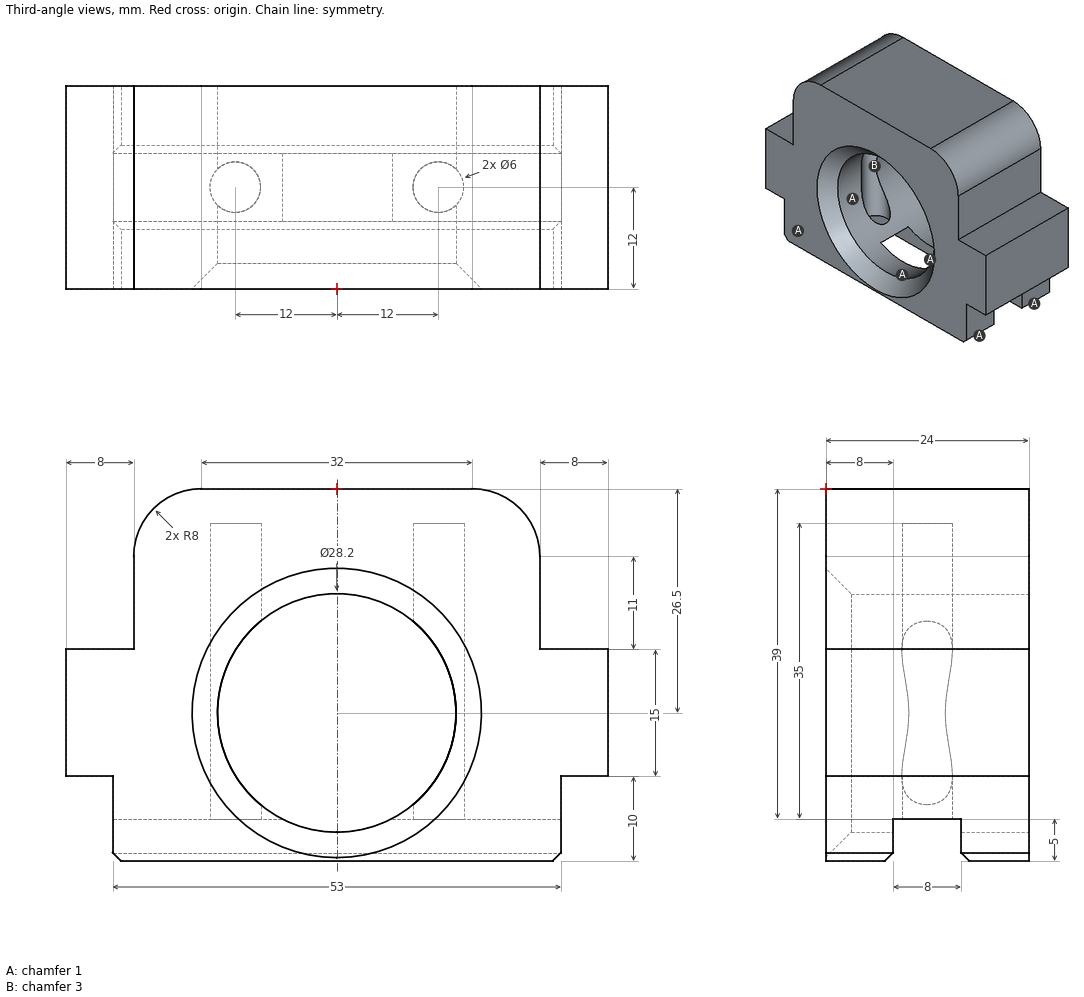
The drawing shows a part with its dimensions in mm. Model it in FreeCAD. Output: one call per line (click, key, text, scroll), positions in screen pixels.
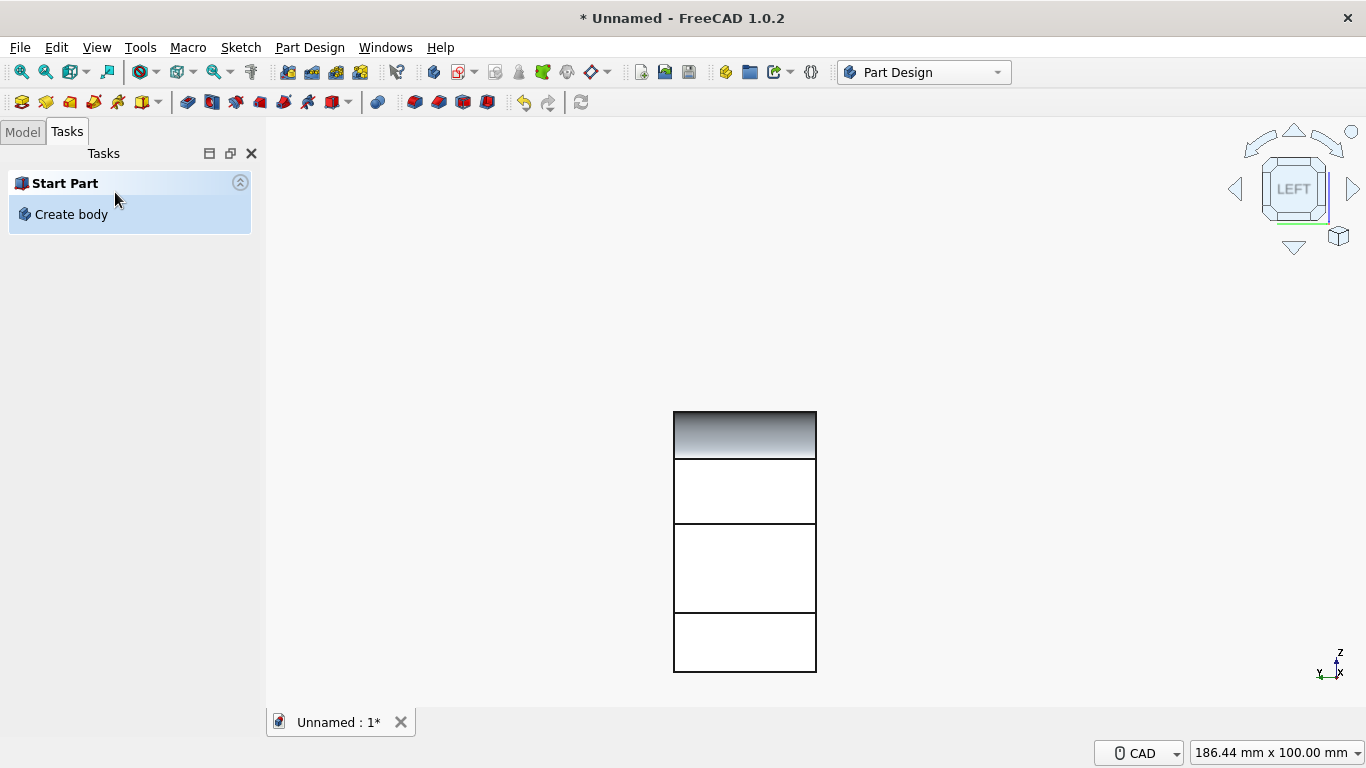
click(22, 72)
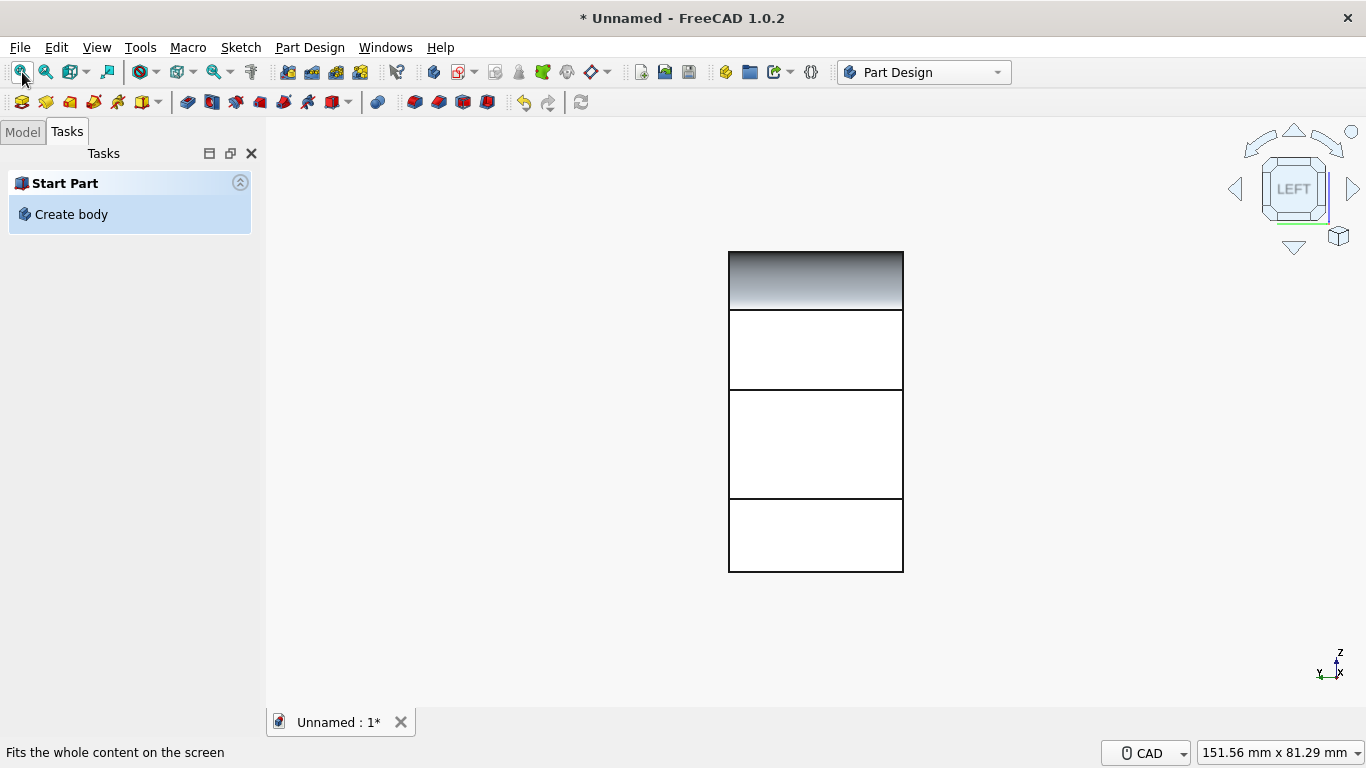
click(766, 534)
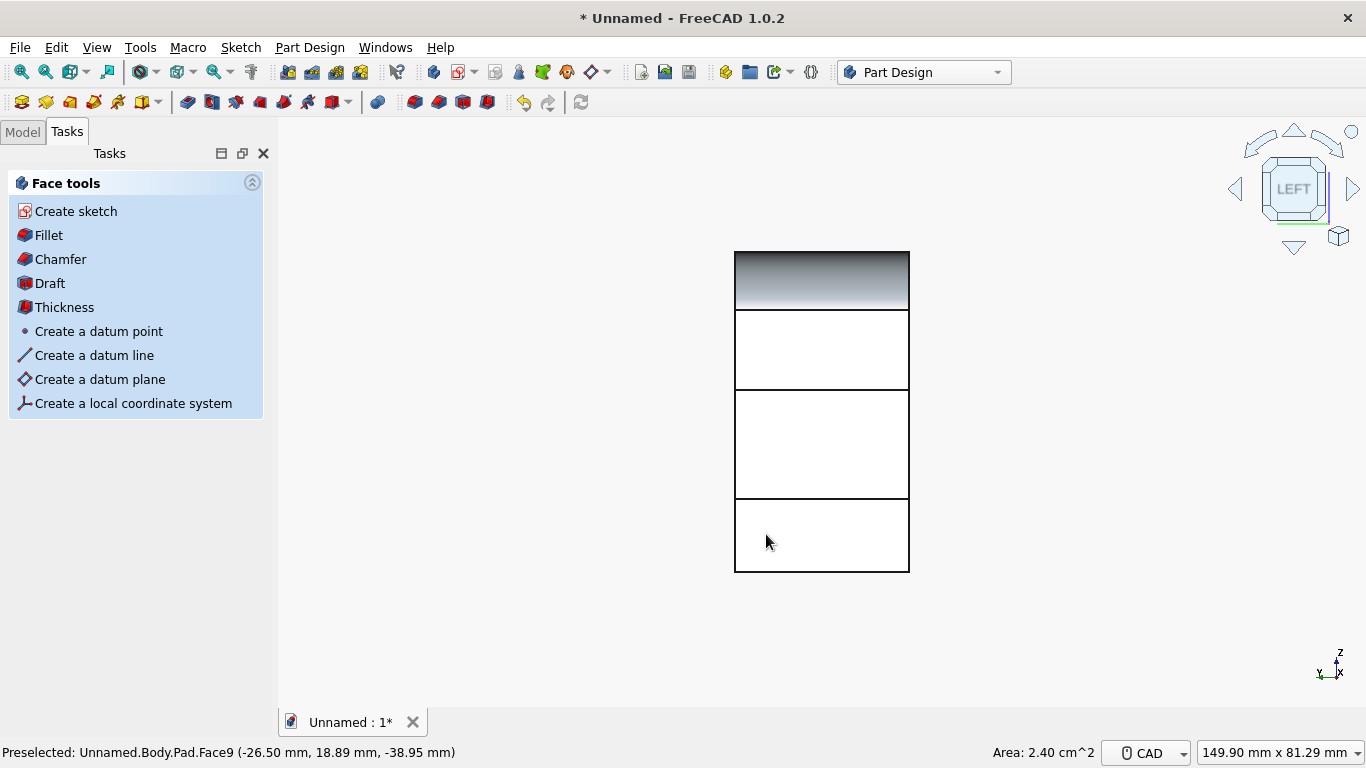
click(458, 72)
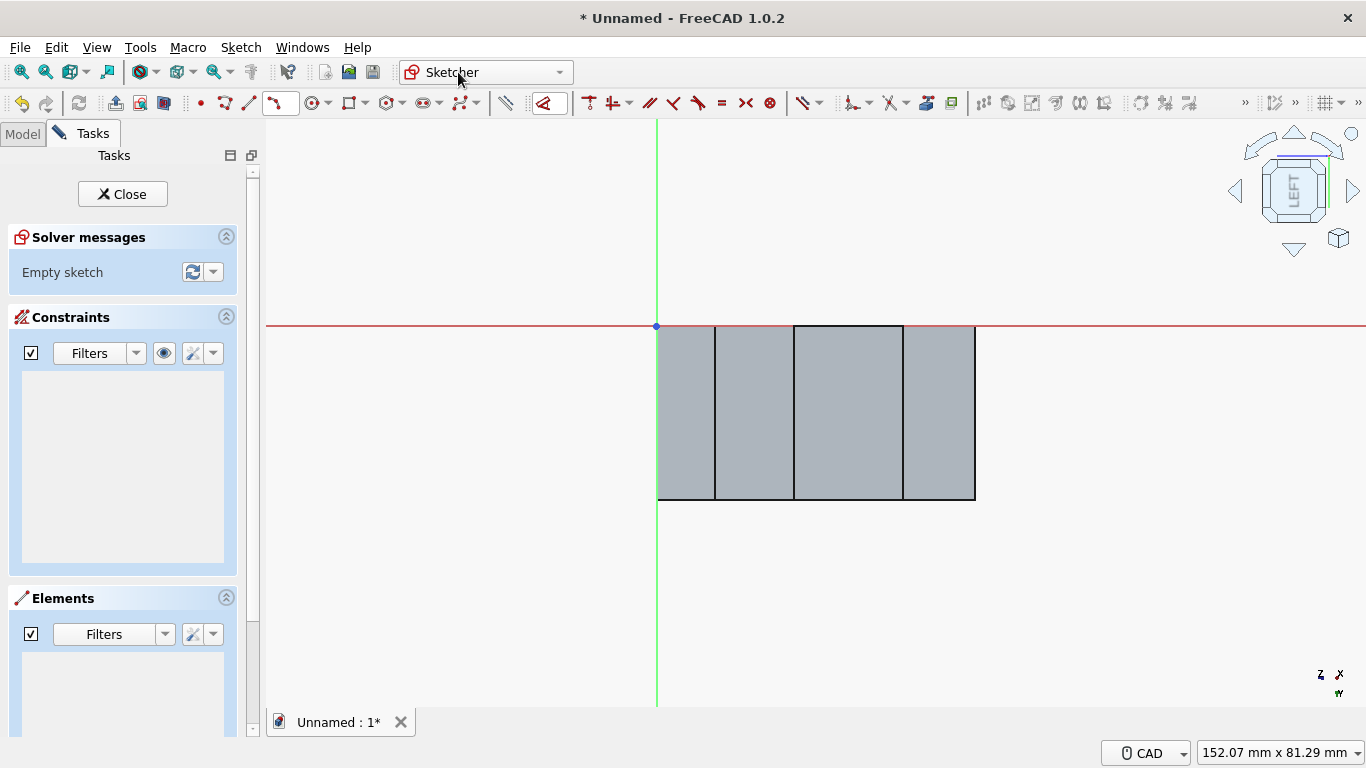
click(164, 104)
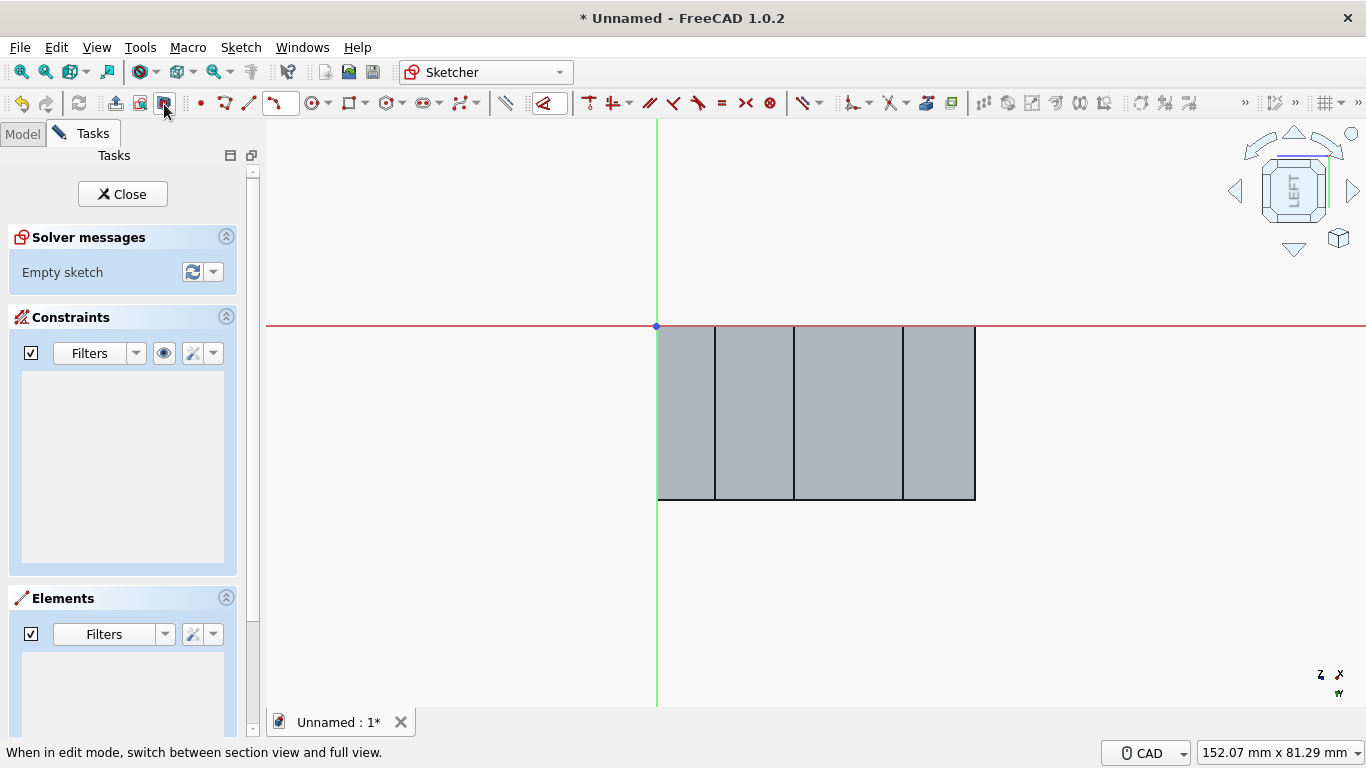
scroll(999, 413, up, 9)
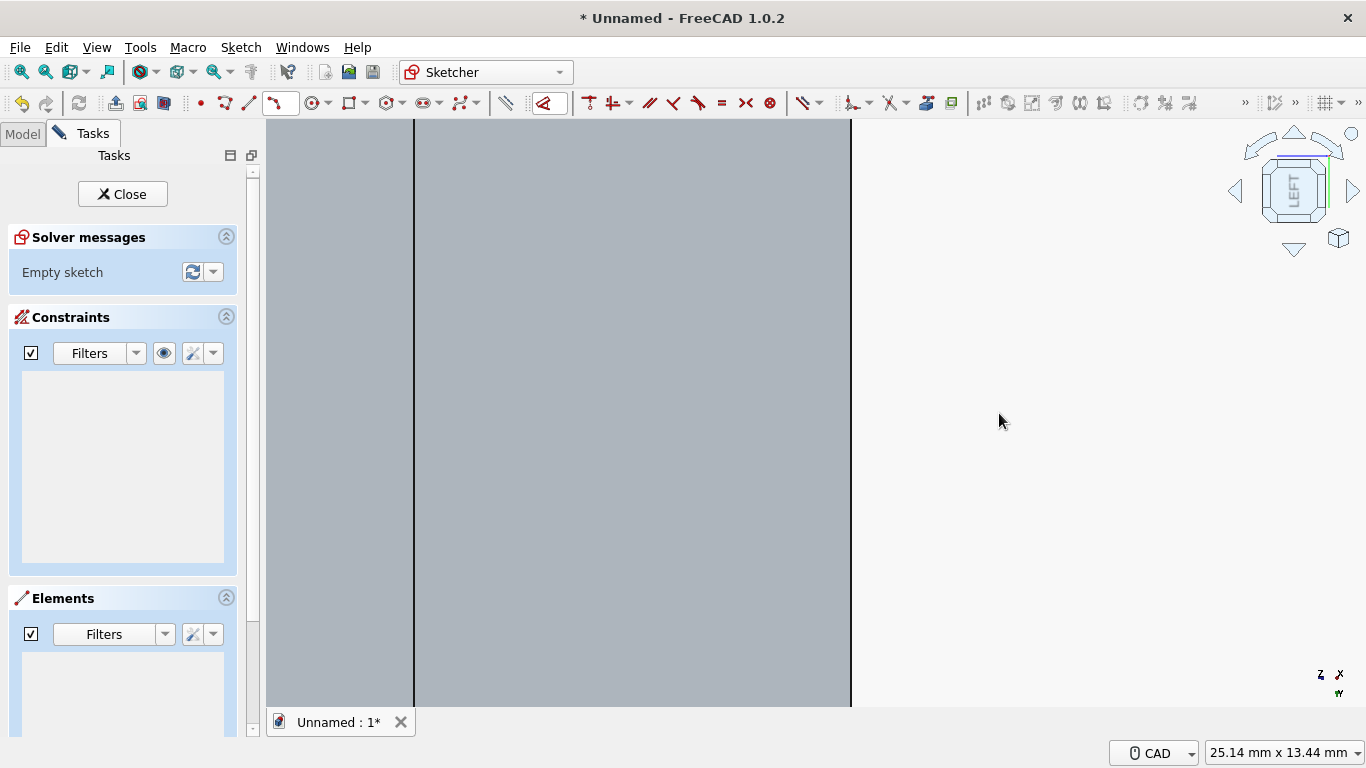
click(350, 104)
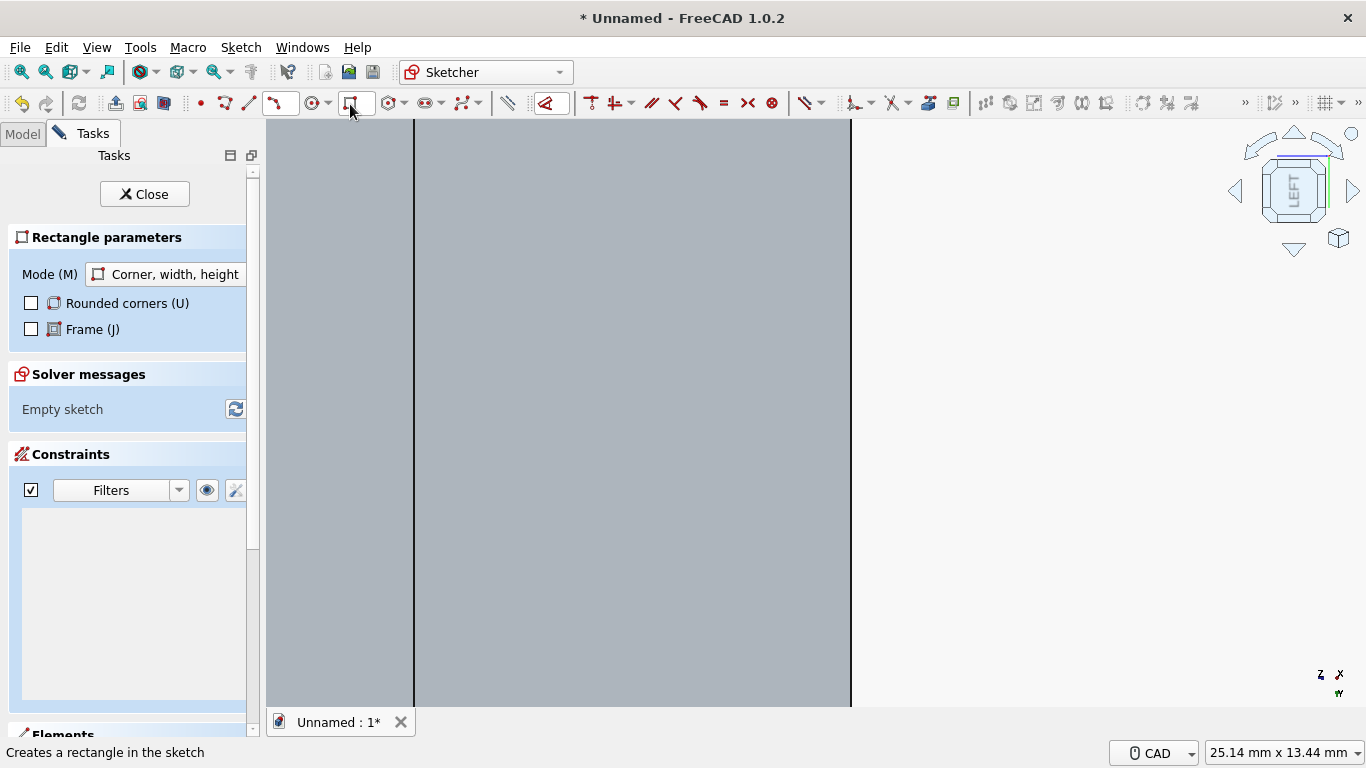
click(632, 235)
move(851, 586)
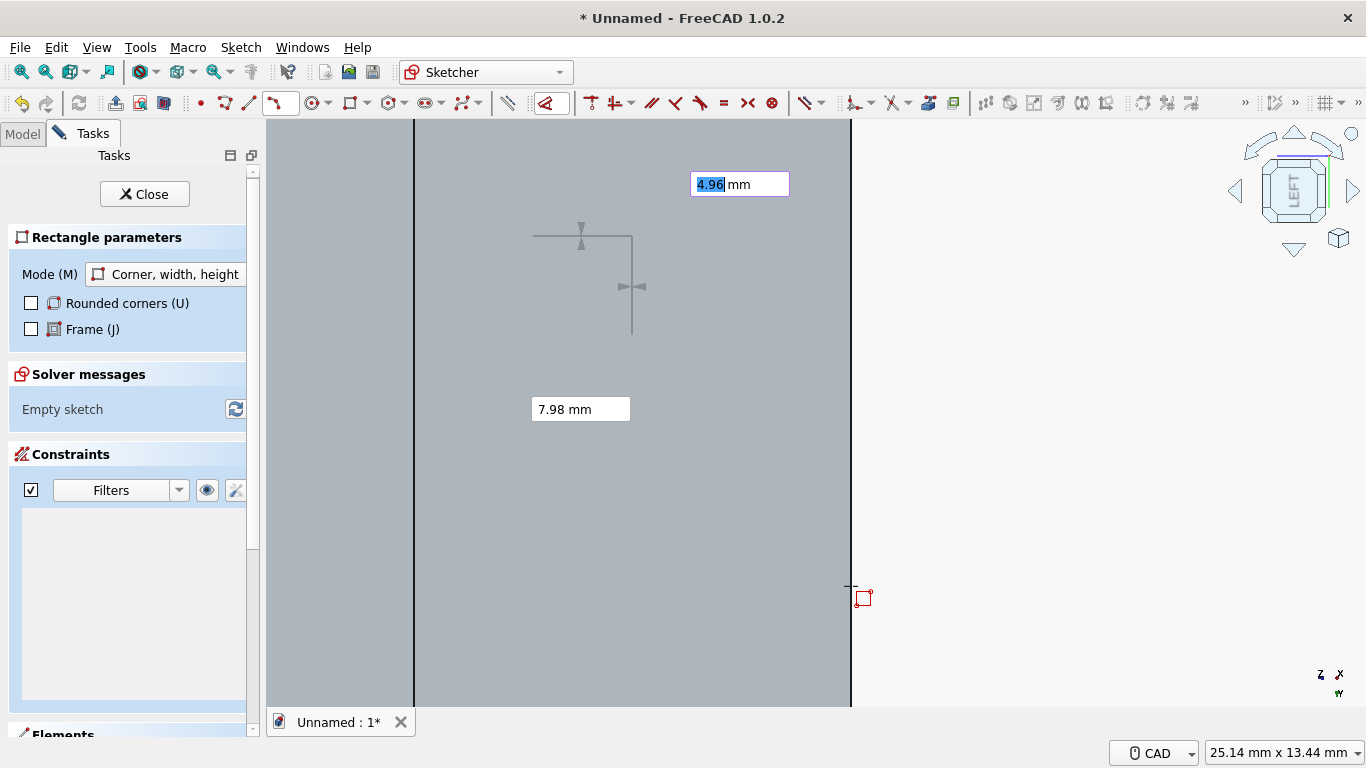
text(5)
key(Tab)
text(8)
key(Return)
key(Escape)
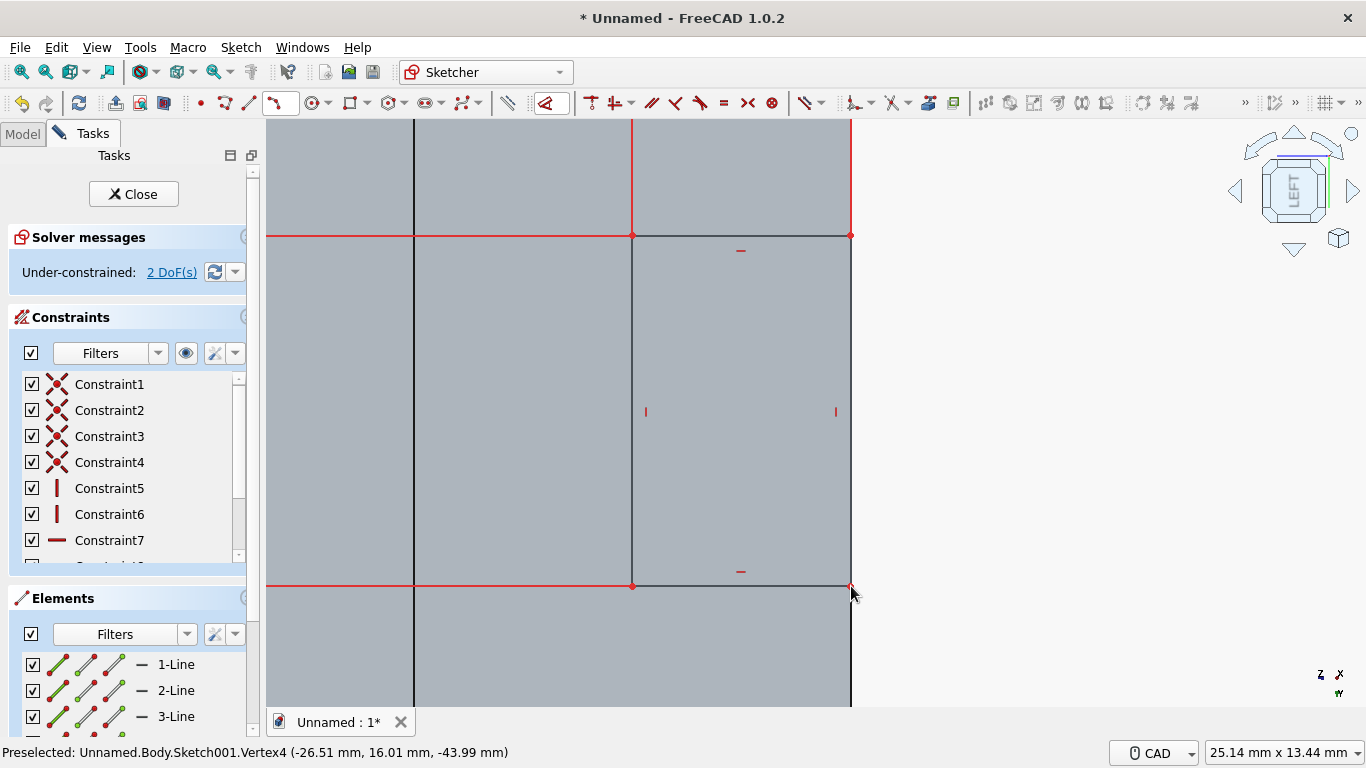
click(632, 236)